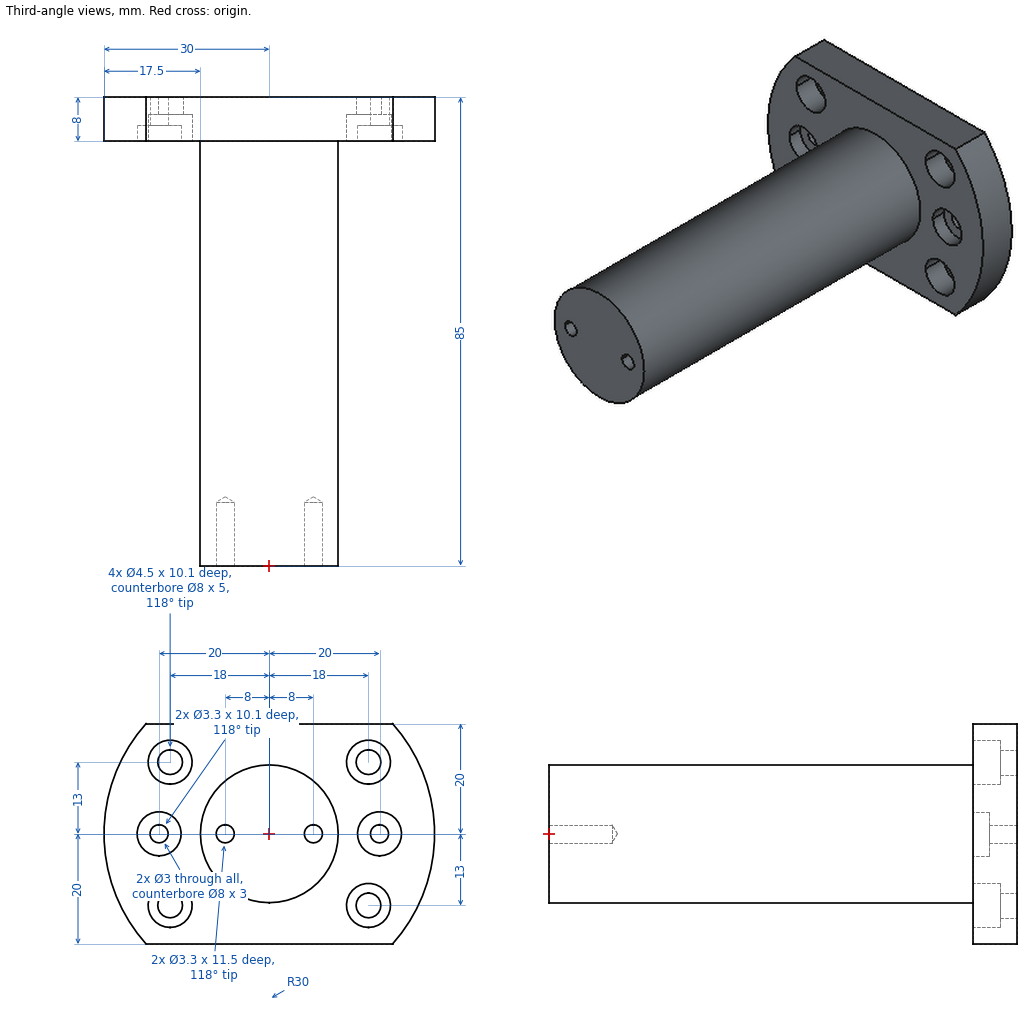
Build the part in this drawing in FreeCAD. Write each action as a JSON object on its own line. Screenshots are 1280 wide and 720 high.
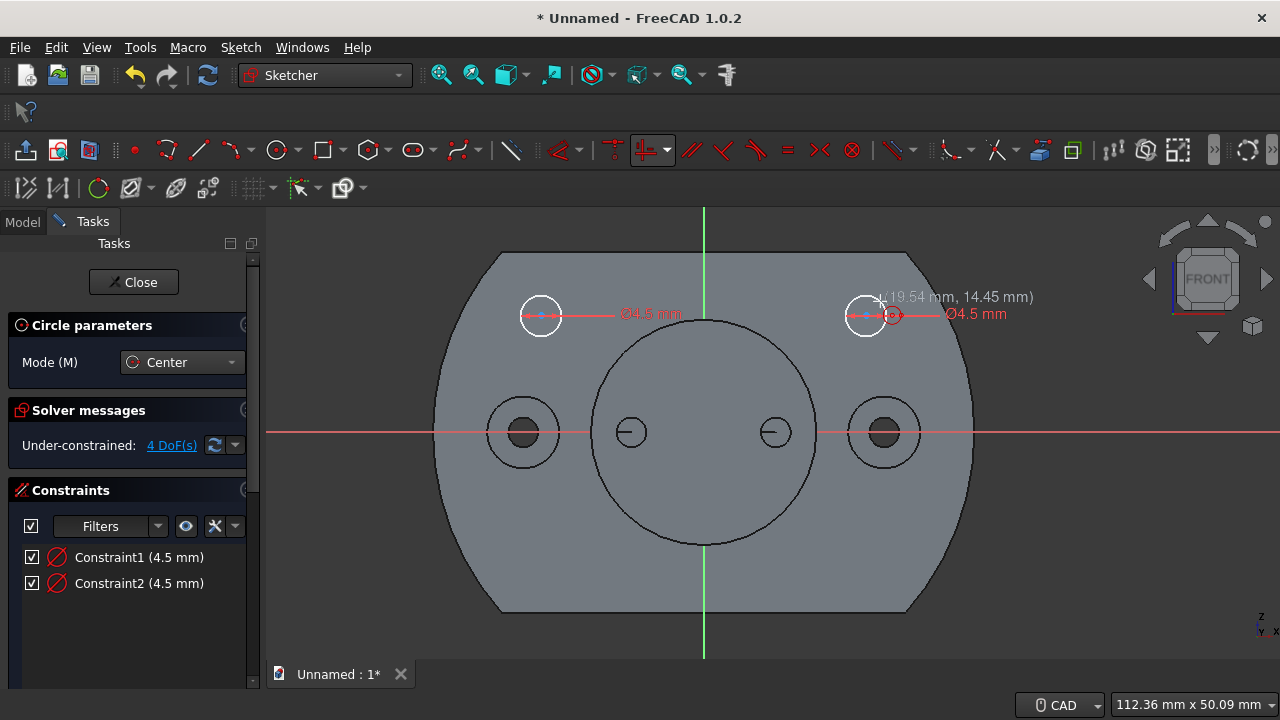
{"action": "left_click", "coordinate": [866, 550]}
{"action": "mouse_move", "coordinate": [880, 535]}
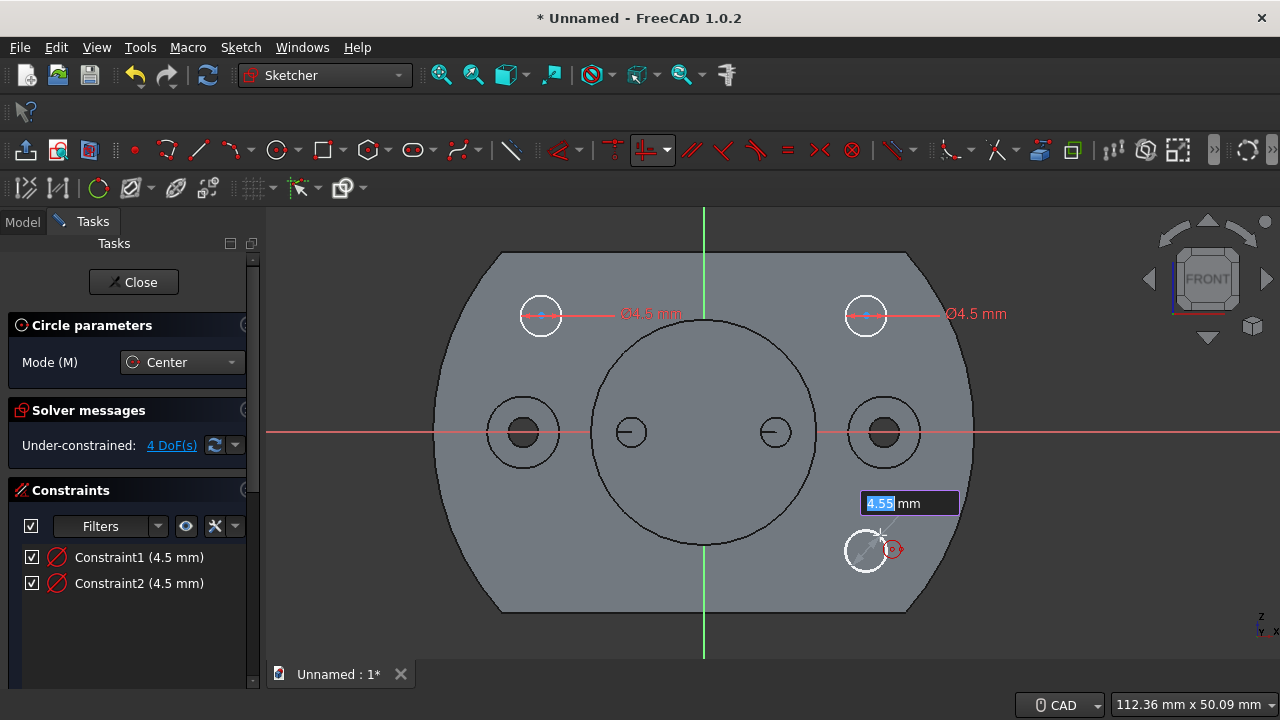
{"action": "type", "text": "4.5"}
{"action": "key", "text": "Return"}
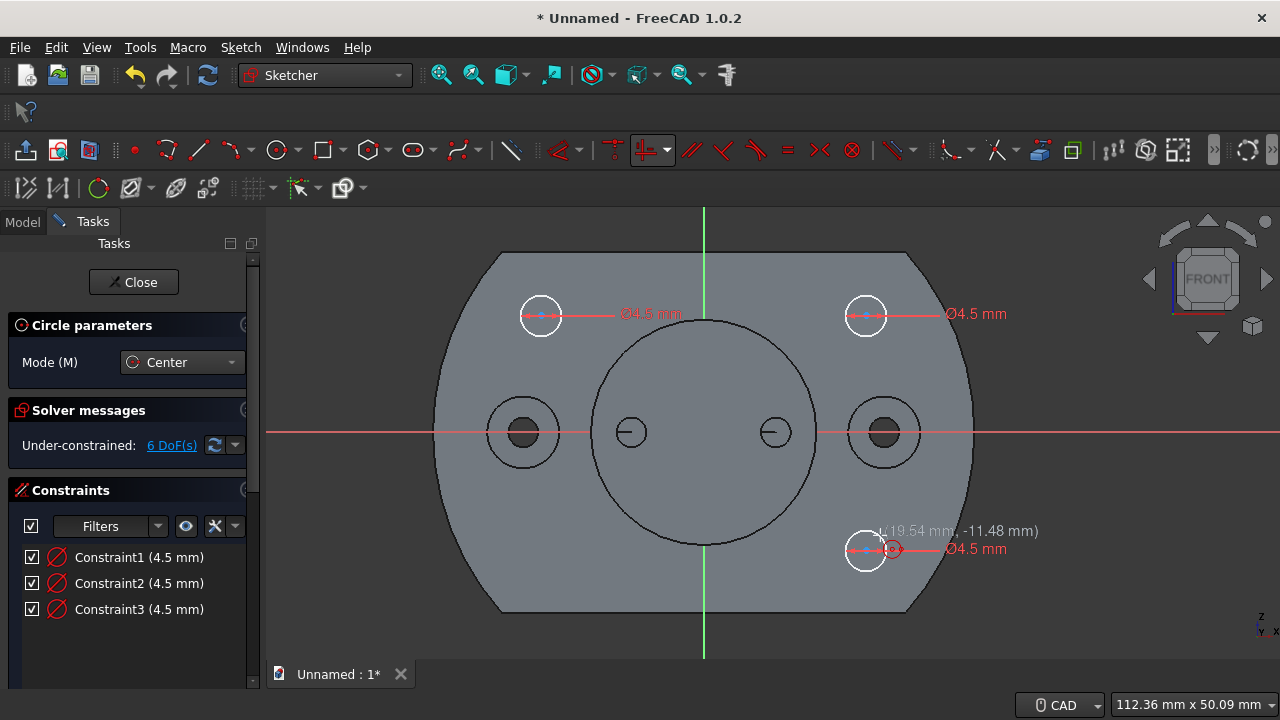
{"action": "left_click", "coordinate": [541, 550]}
{"action": "mouse_move", "coordinate": [556, 535]}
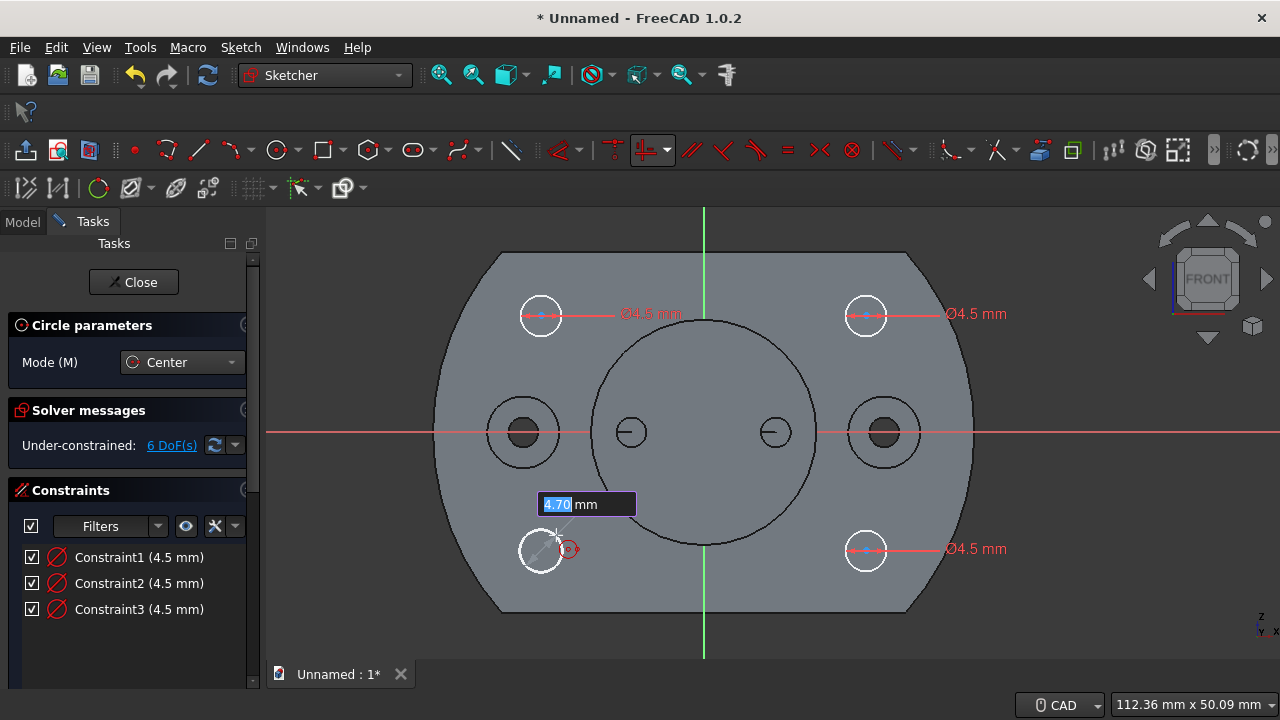
{"action": "type", "text": "4.5"}
{"action": "key", "text": "Return"}
{"action": "key", "text": "Escape"}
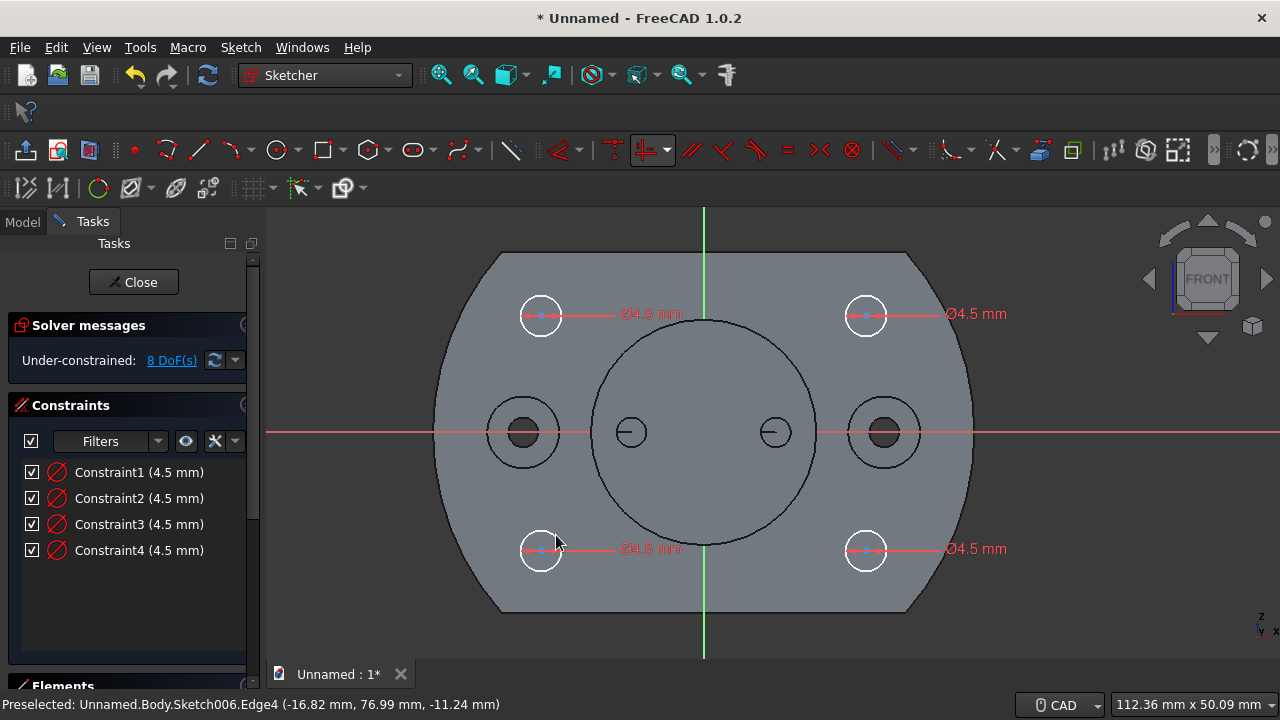
{"action": "left_click", "coordinate": [541, 316]}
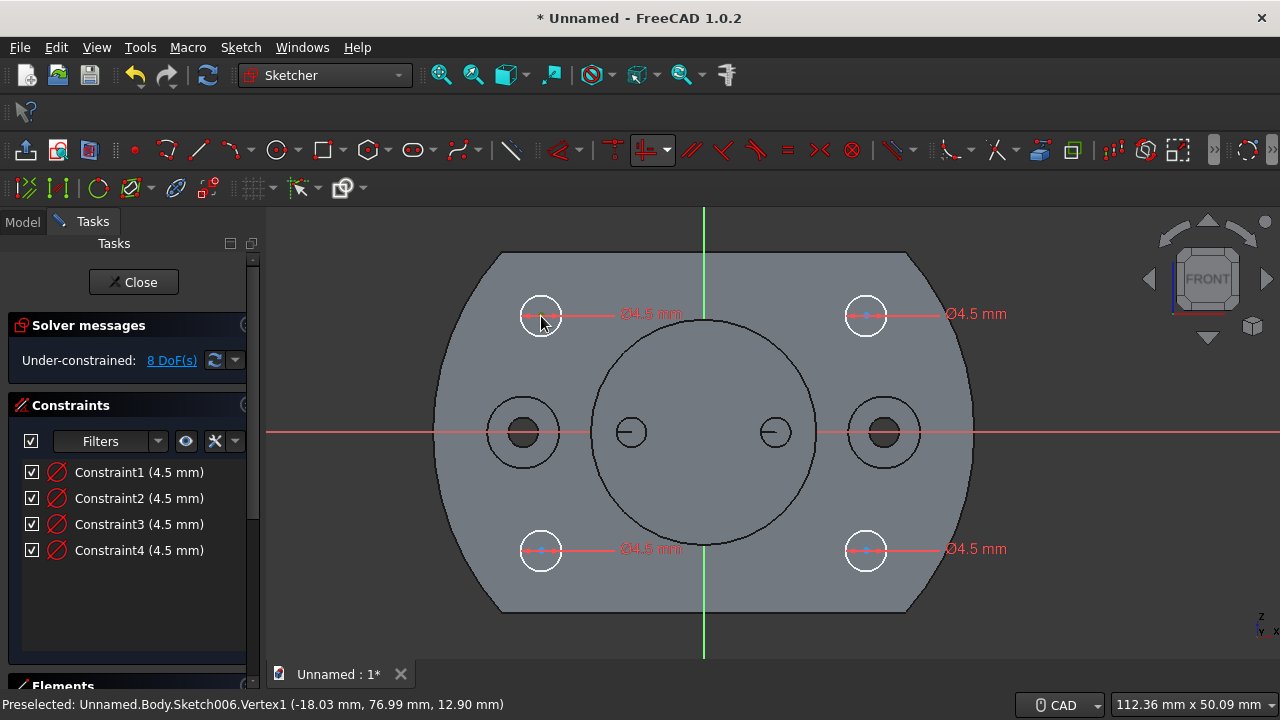
{"action": "left_click", "coordinate": [866, 316]}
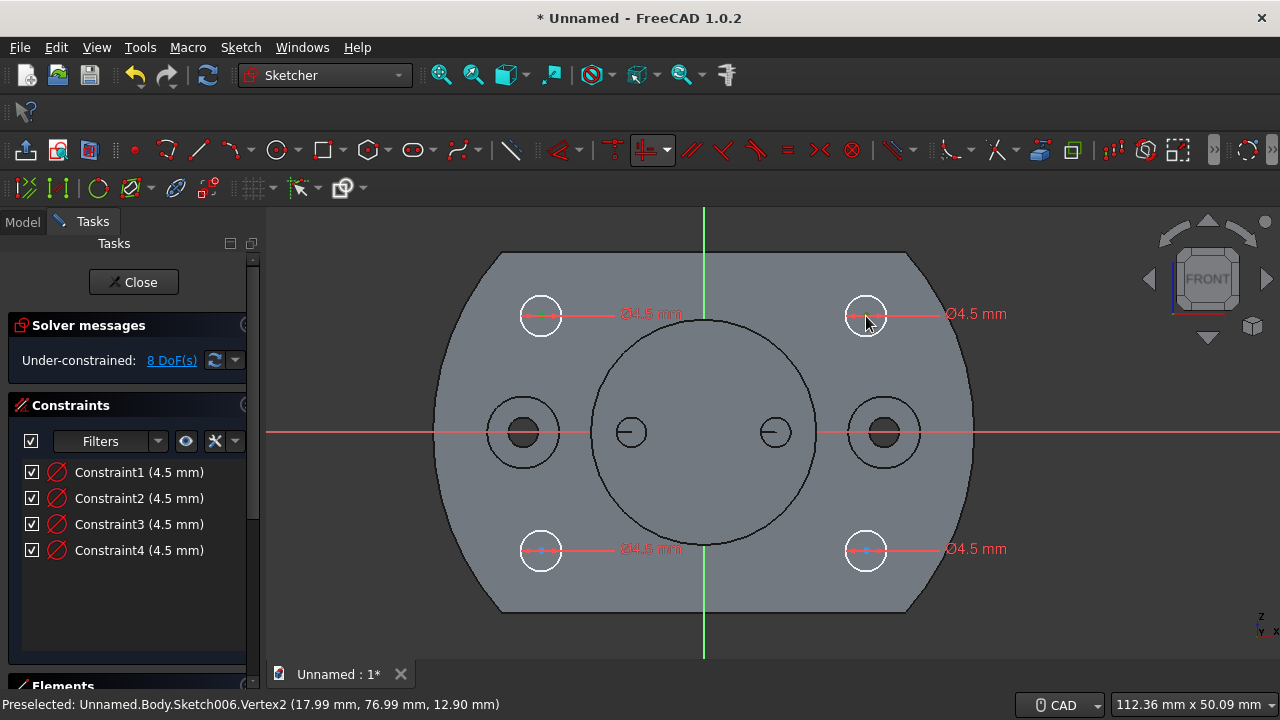
{"action": "left_click", "coordinate": [670, 150]}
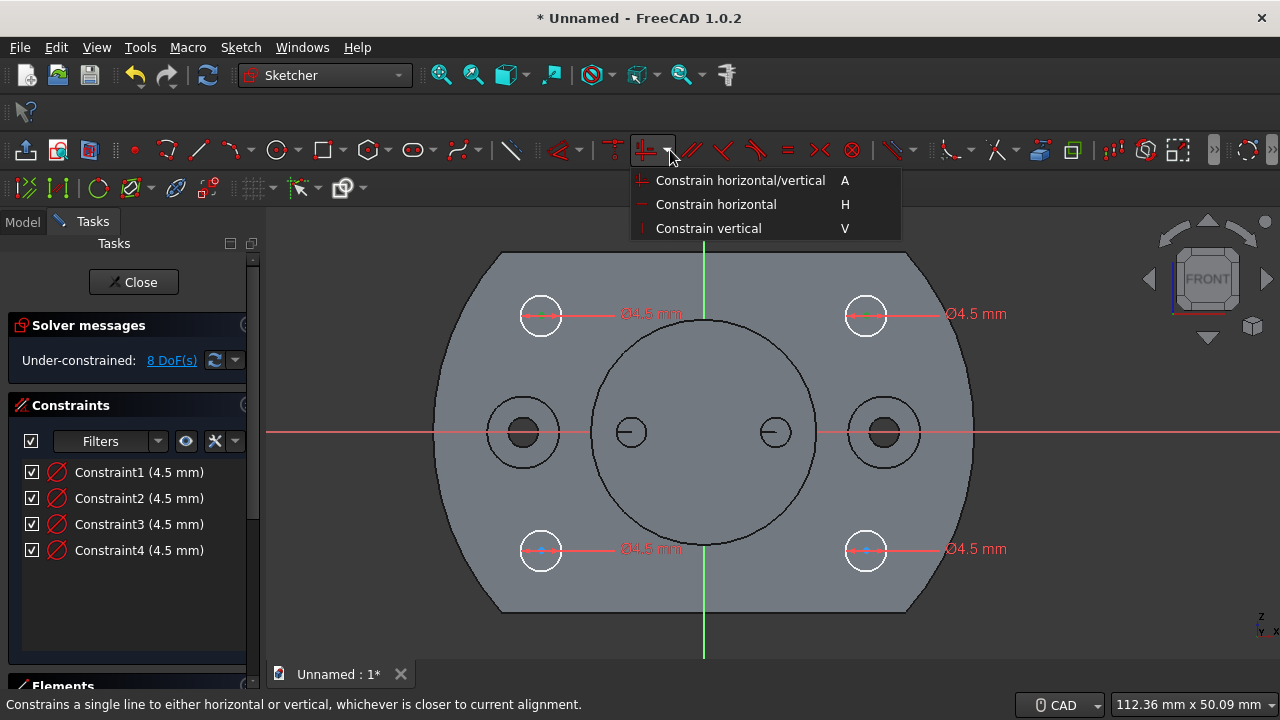
{"action": "left_click", "coordinate": [766, 204]}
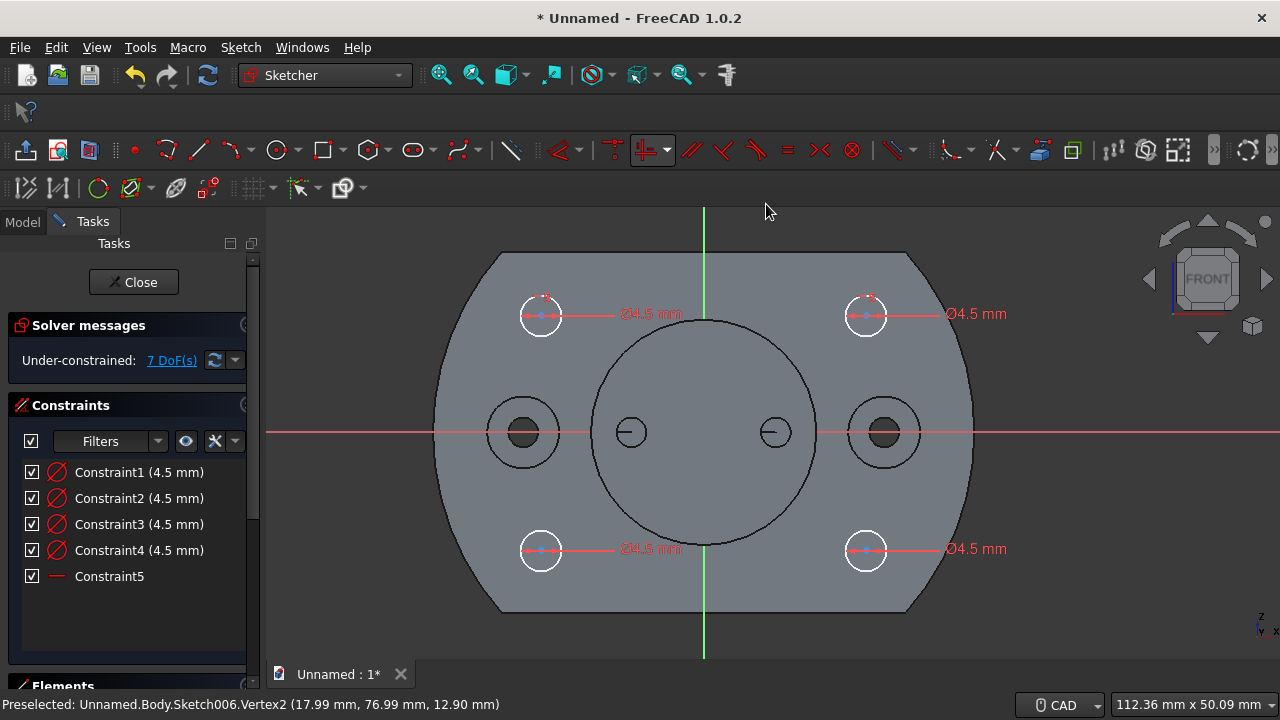
{"action": "left_click", "coordinate": [866, 316]}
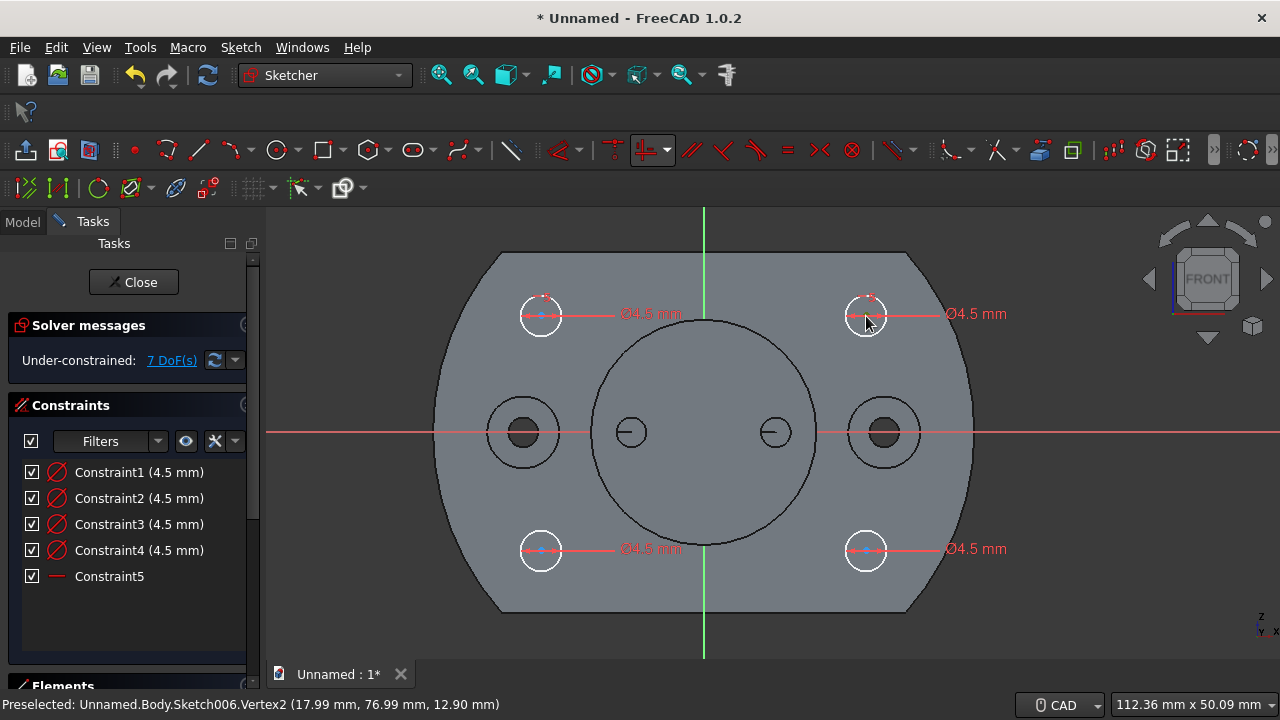
{"action": "left_click", "coordinate": [866, 551]}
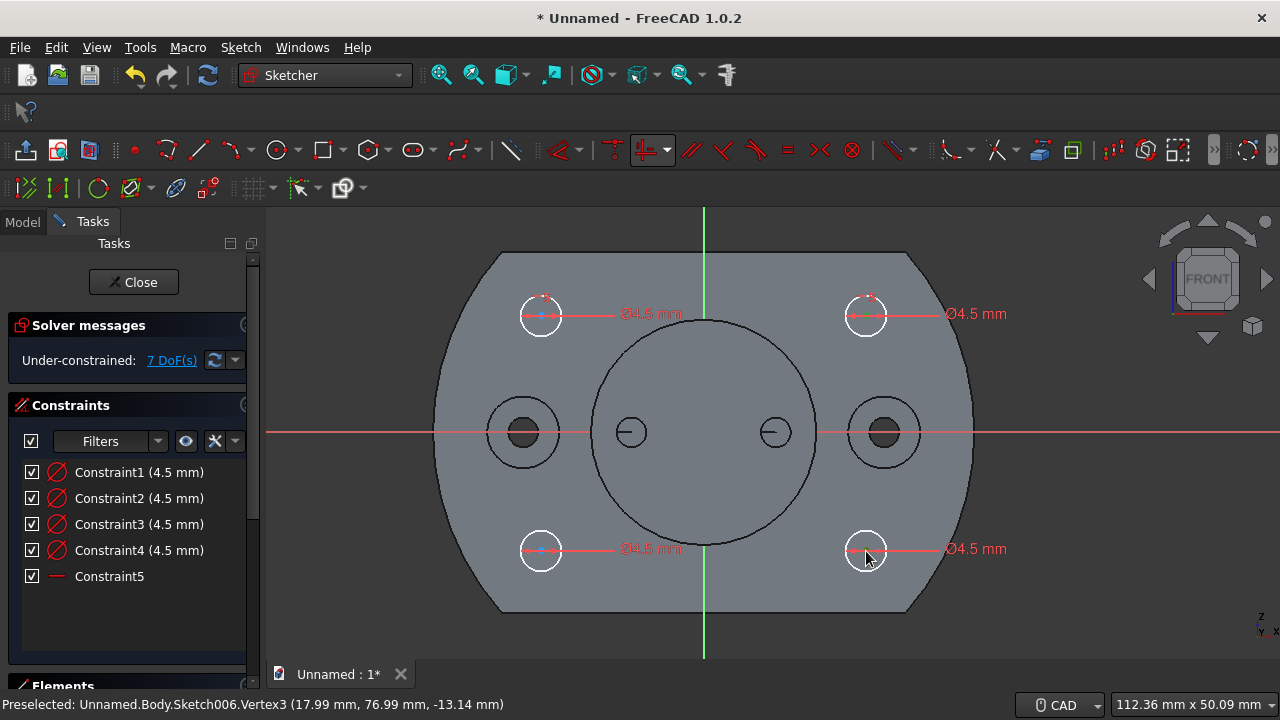
{"action": "left_click", "coordinate": [670, 150]}